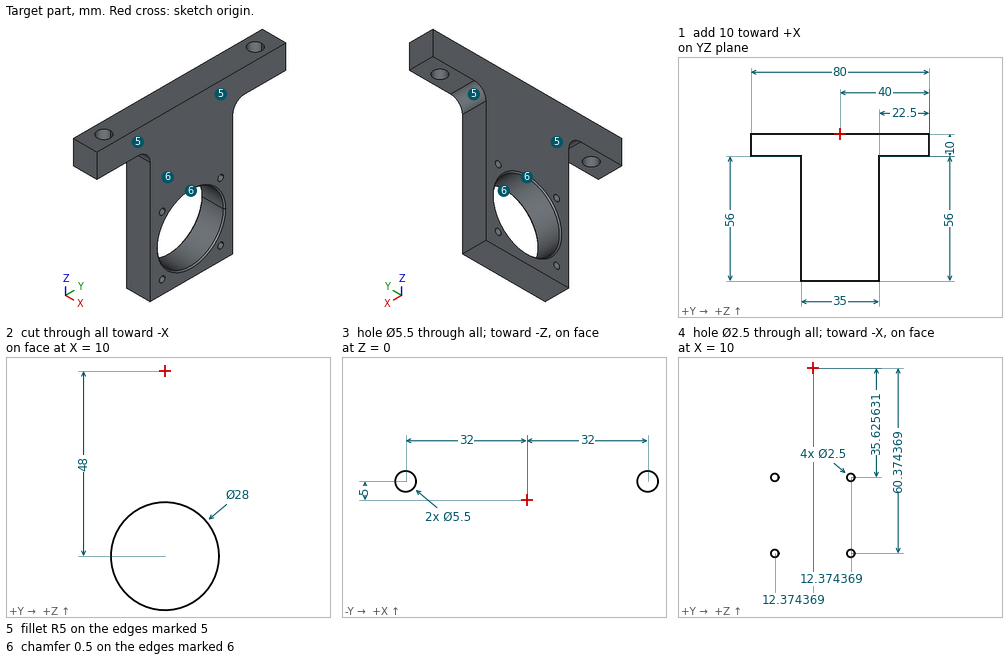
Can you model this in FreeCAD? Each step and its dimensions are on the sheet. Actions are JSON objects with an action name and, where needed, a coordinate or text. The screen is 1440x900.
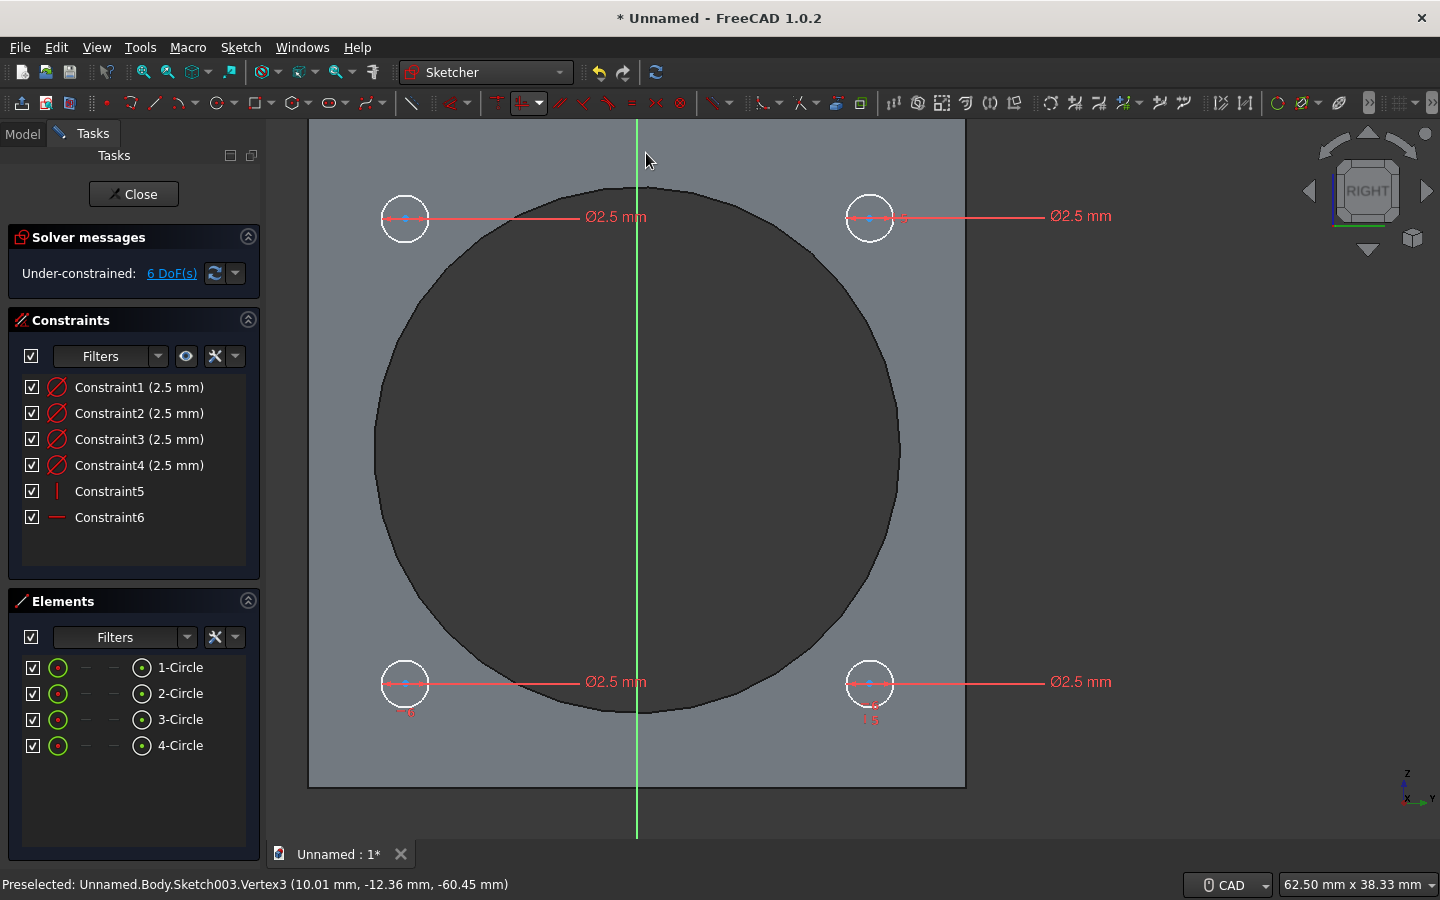
{"action": "left_click", "coordinate": [405, 684]}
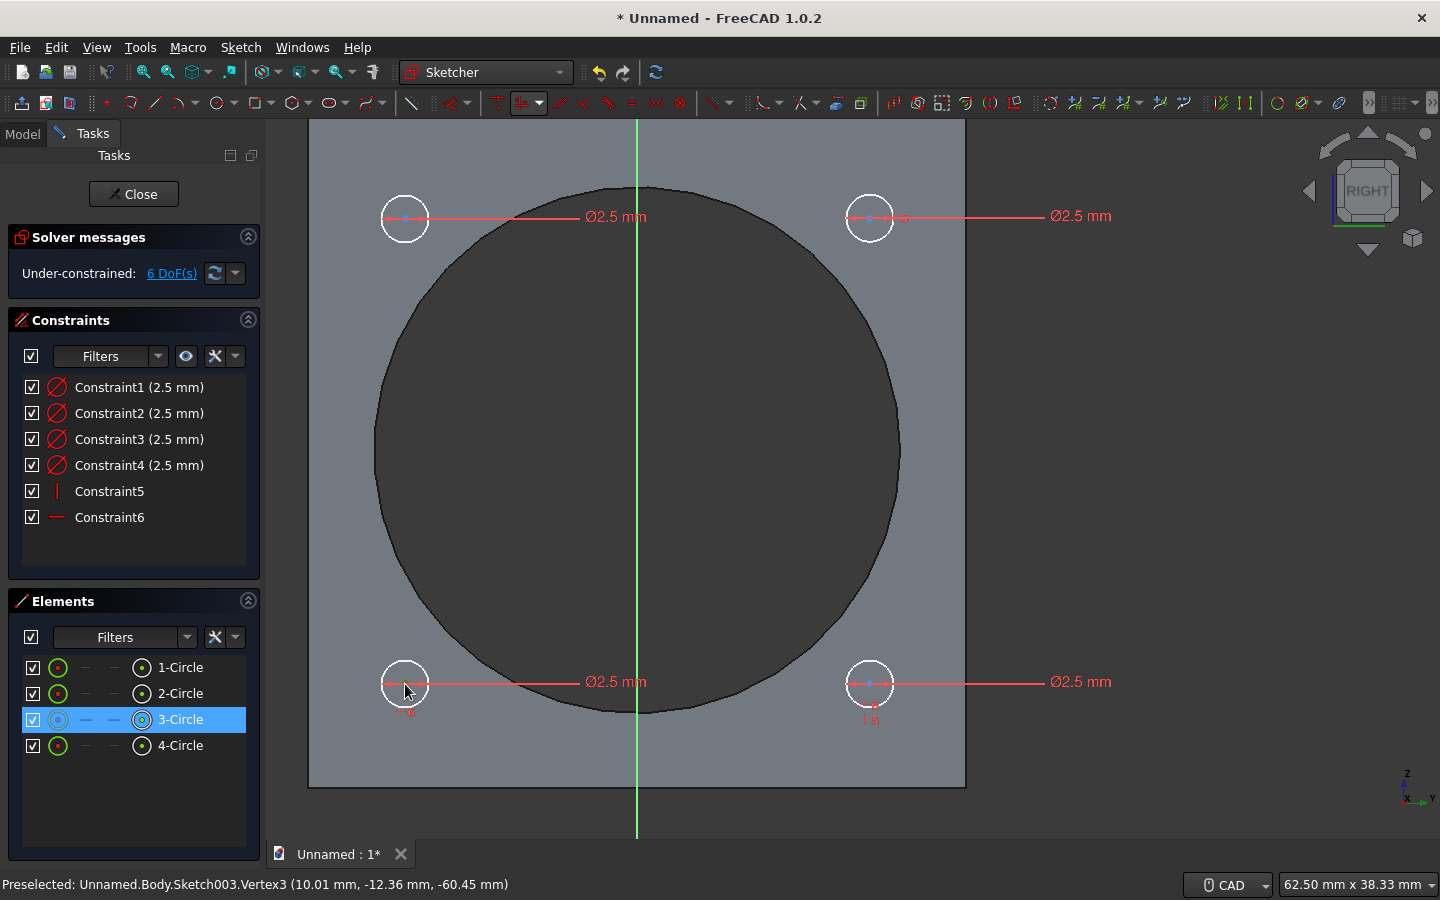
{"action": "left_click", "coordinate": [405, 219]}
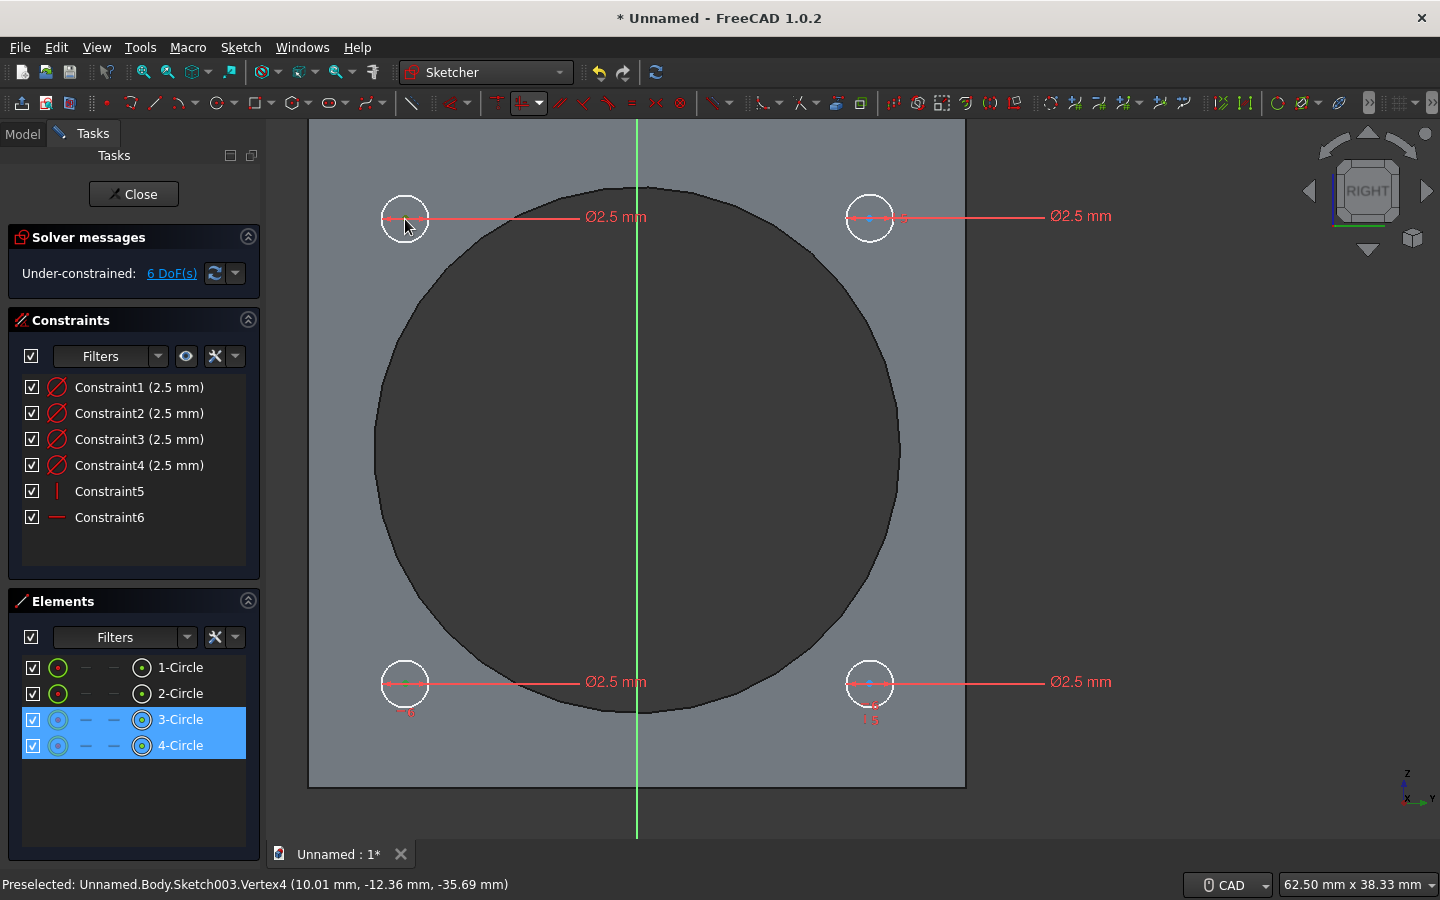
{"action": "key", "text": "v"}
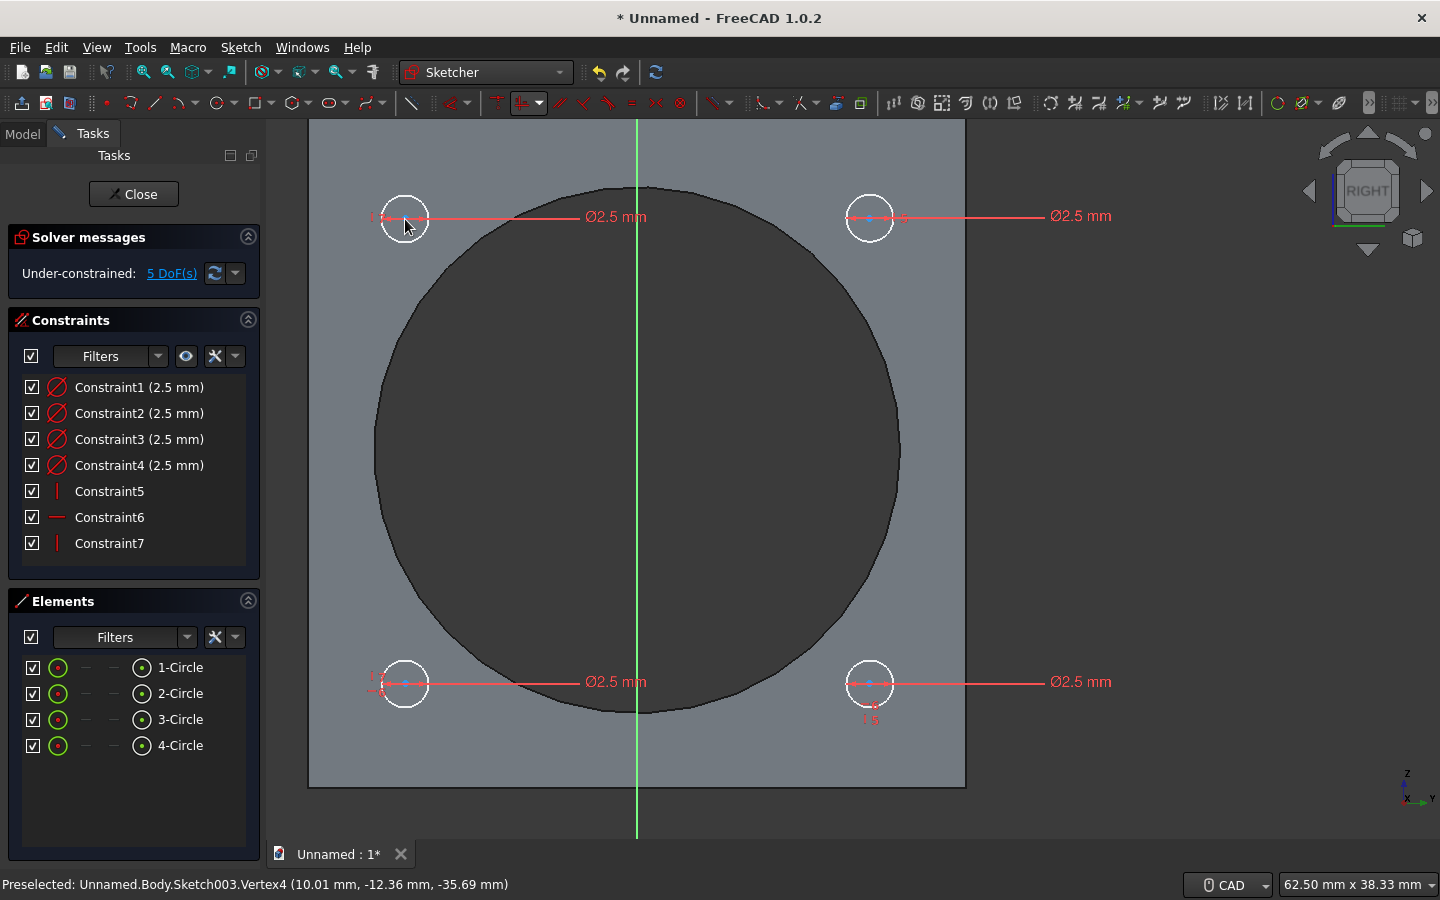
{"action": "left_click", "coordinate": [870, 218]}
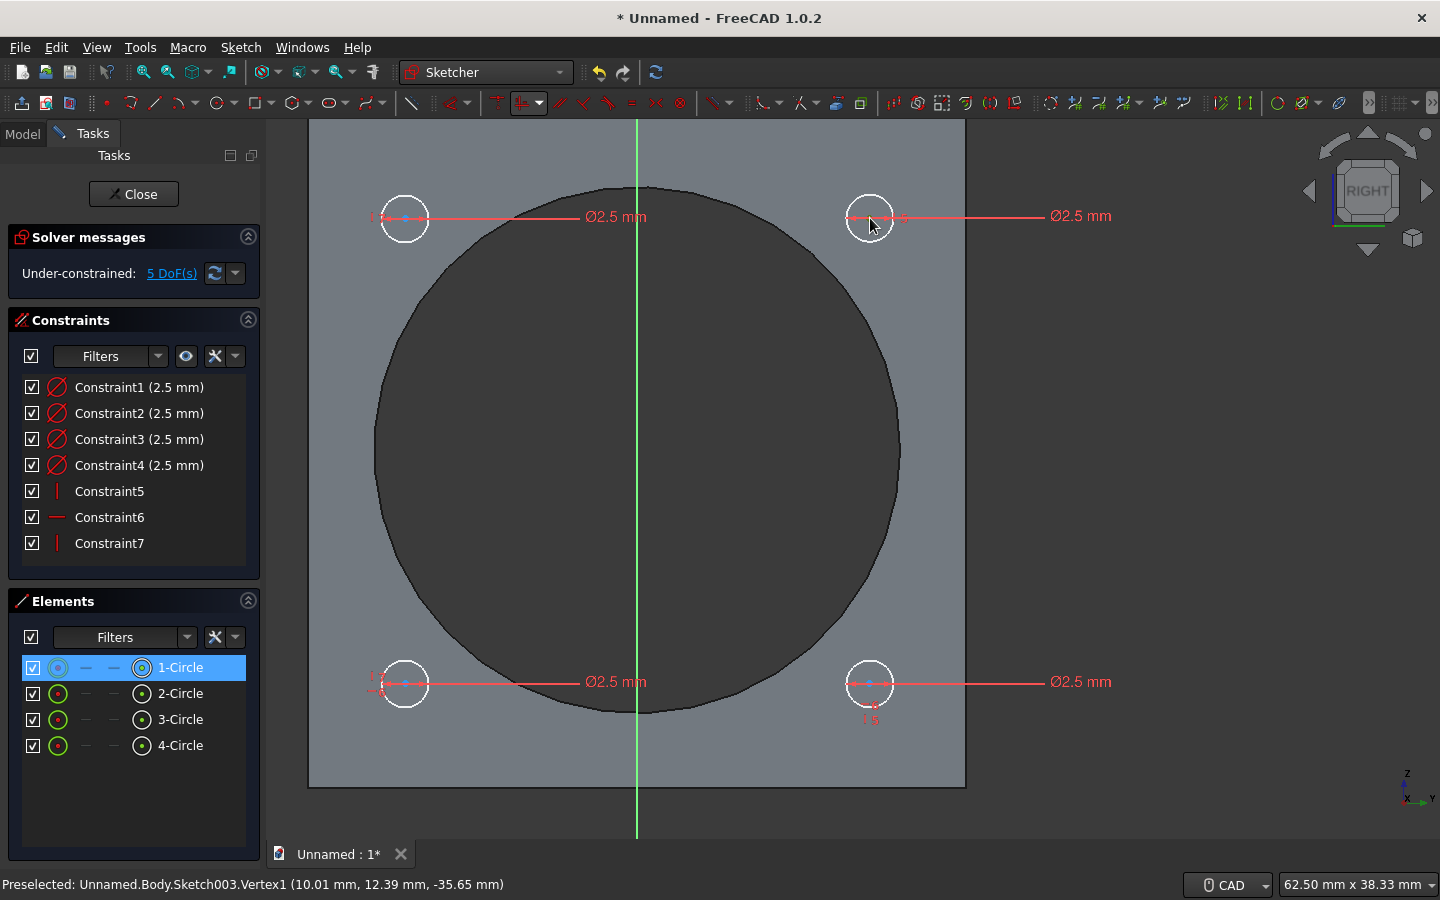
{"action": "left_click", "coordinate": [405, 219]}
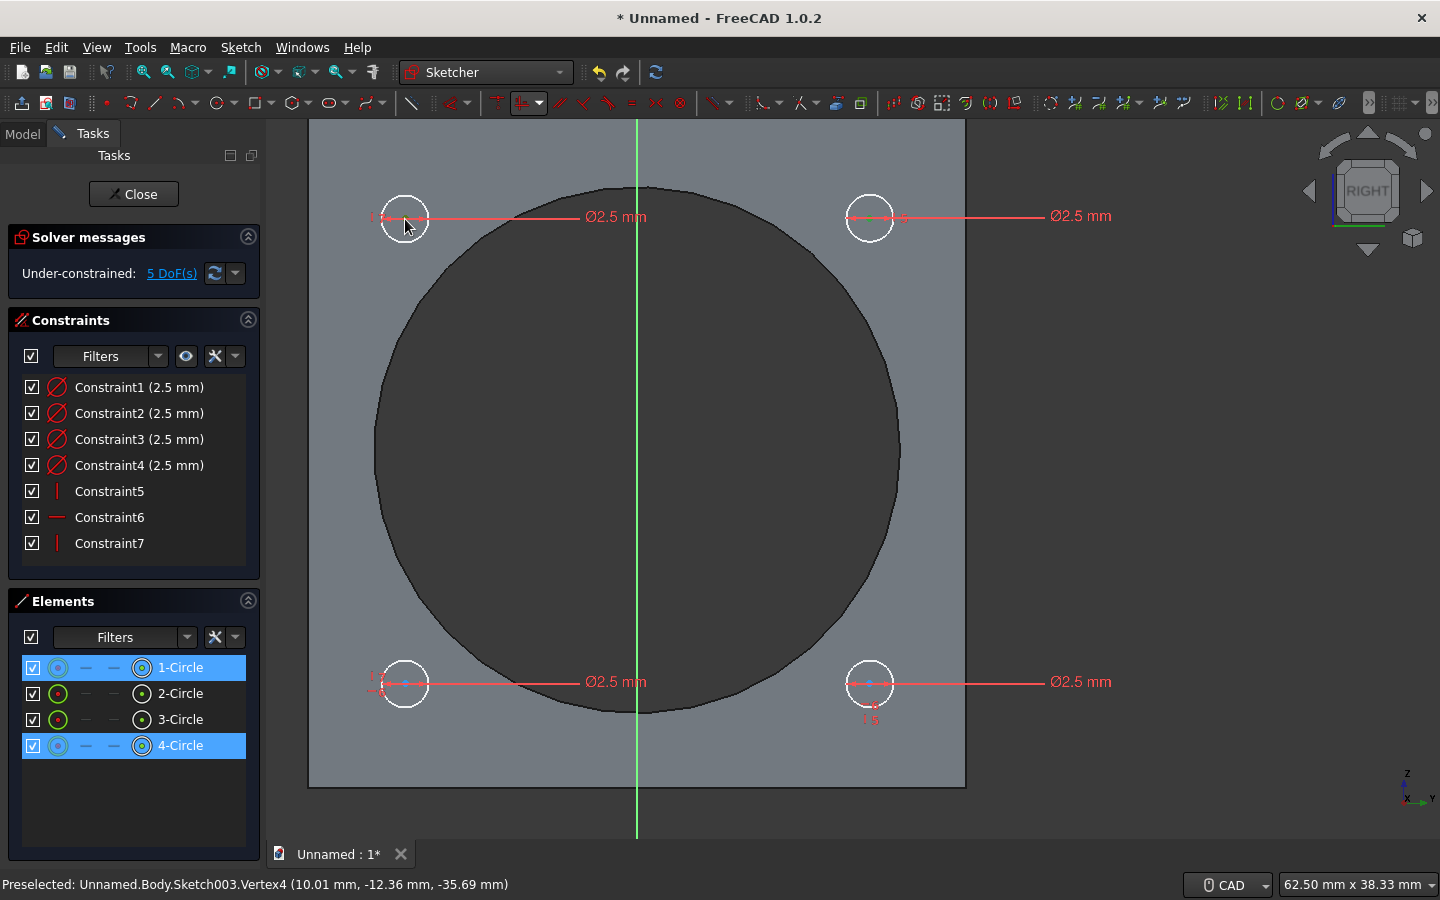
{"action": "left_click", "coordinate": [542, 104]}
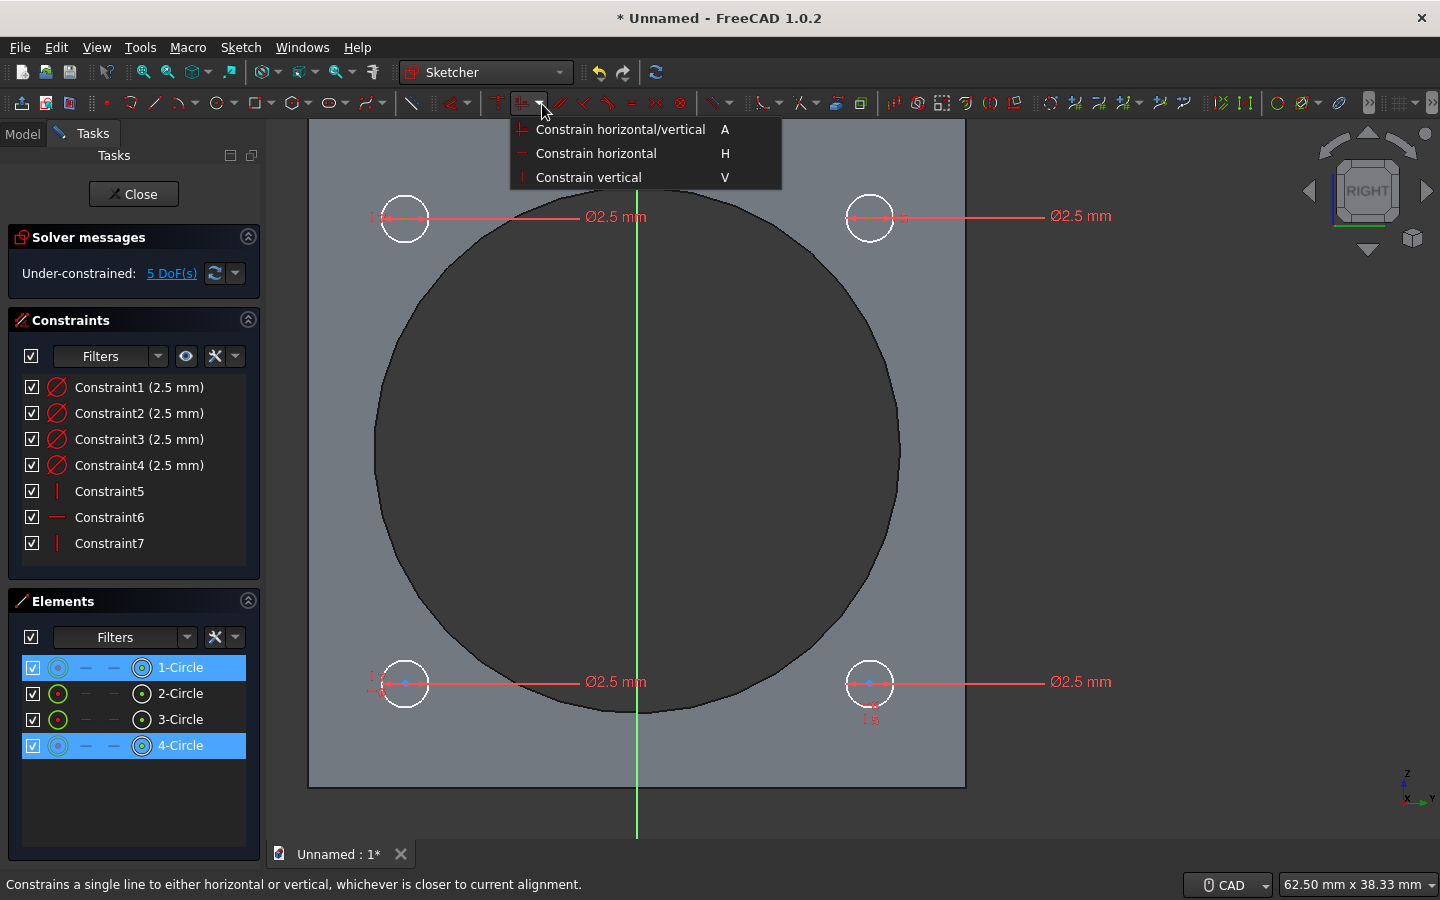
{"action": "left_click", "coordinate": [646, 153]}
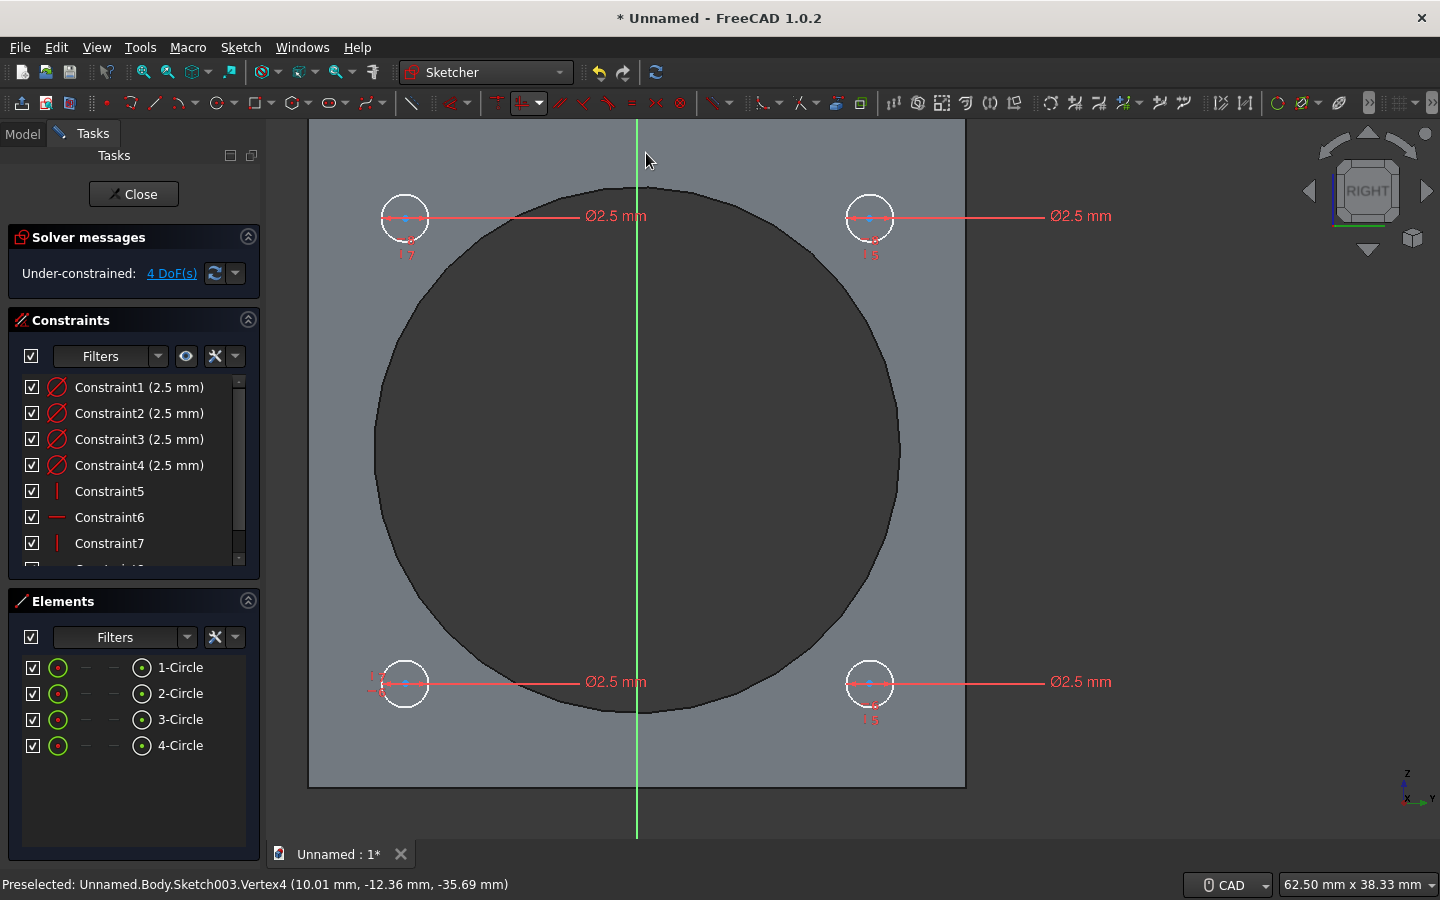
{"action": "left_click", "coordinate": [450, 104]}